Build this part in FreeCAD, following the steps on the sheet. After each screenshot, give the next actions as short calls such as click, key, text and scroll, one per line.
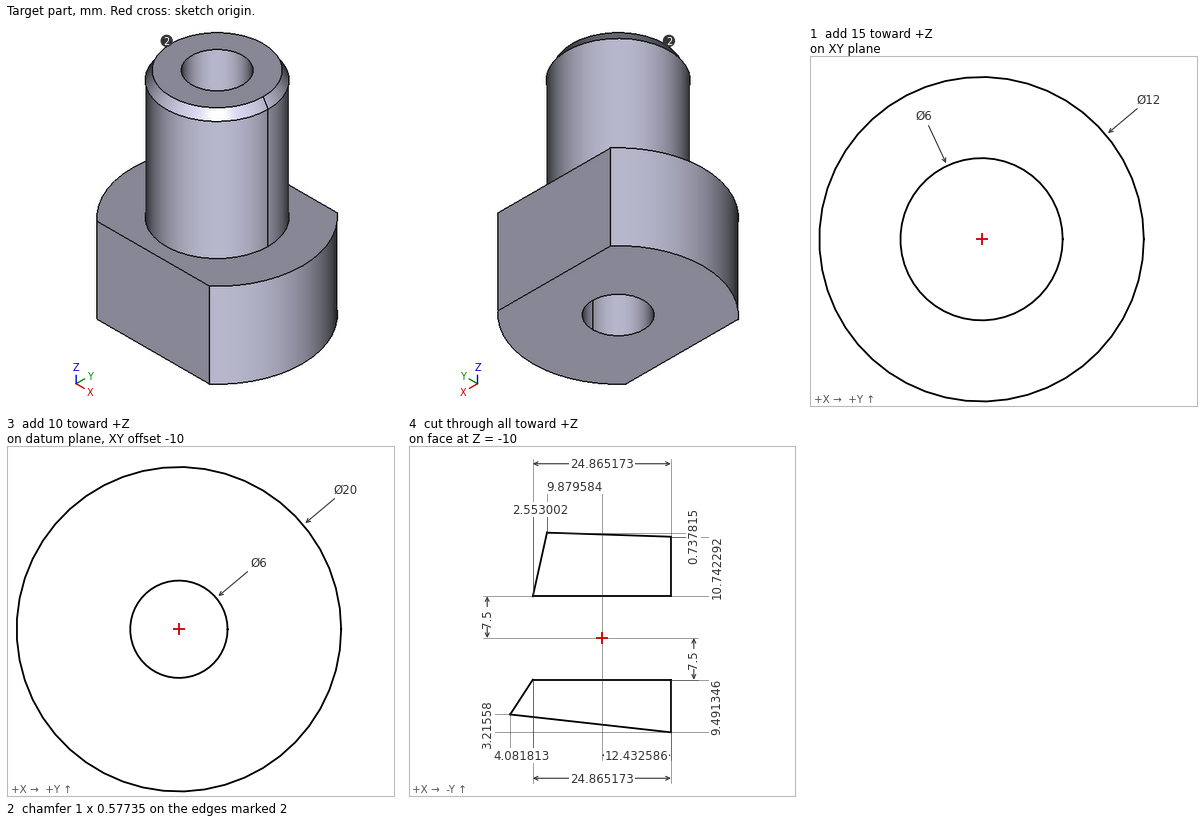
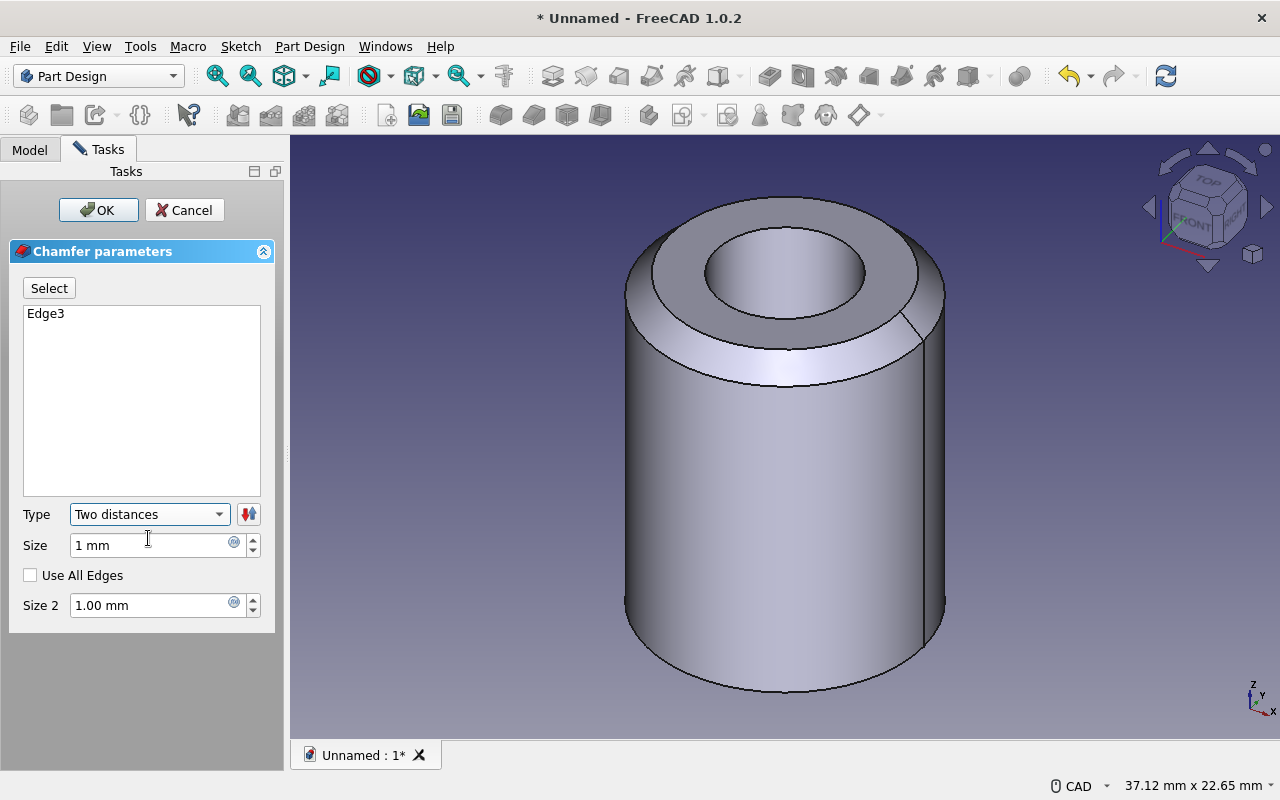
triple_click(158, 606)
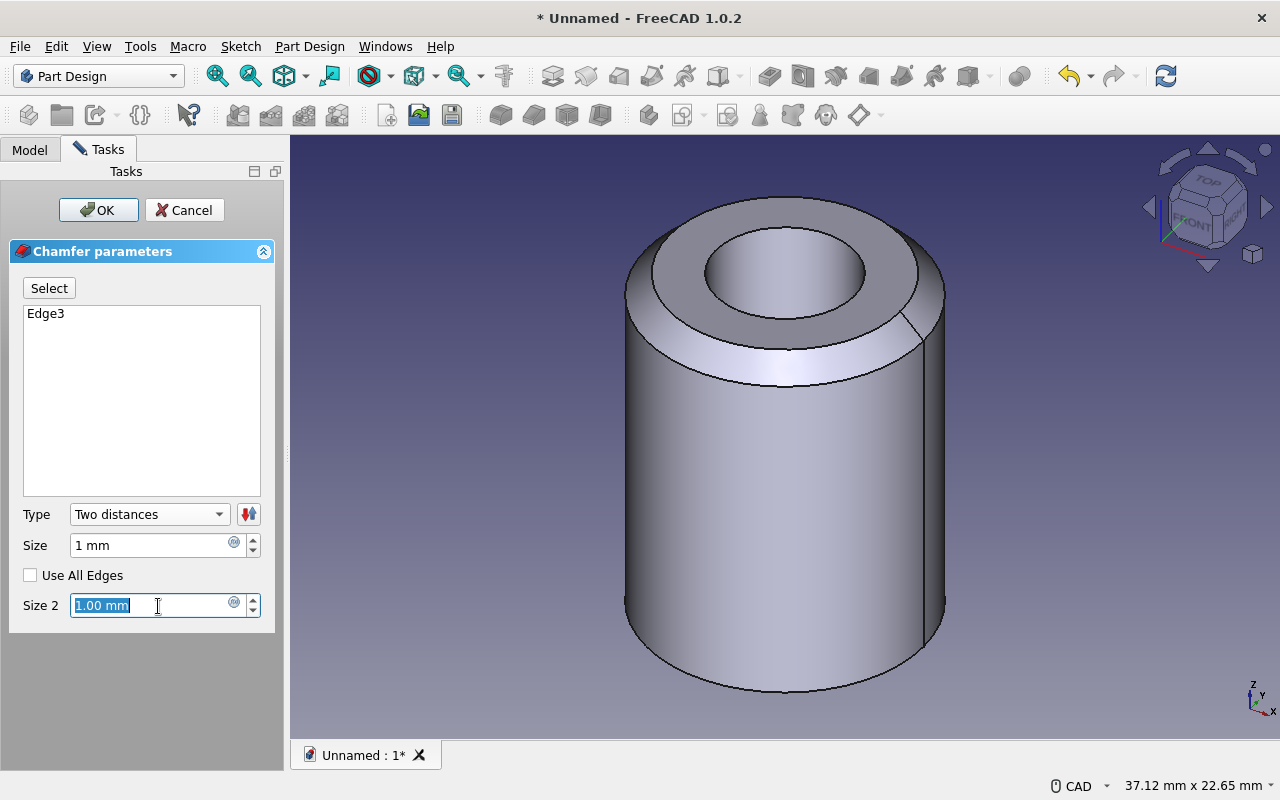
text(0.57735)
key(Tab)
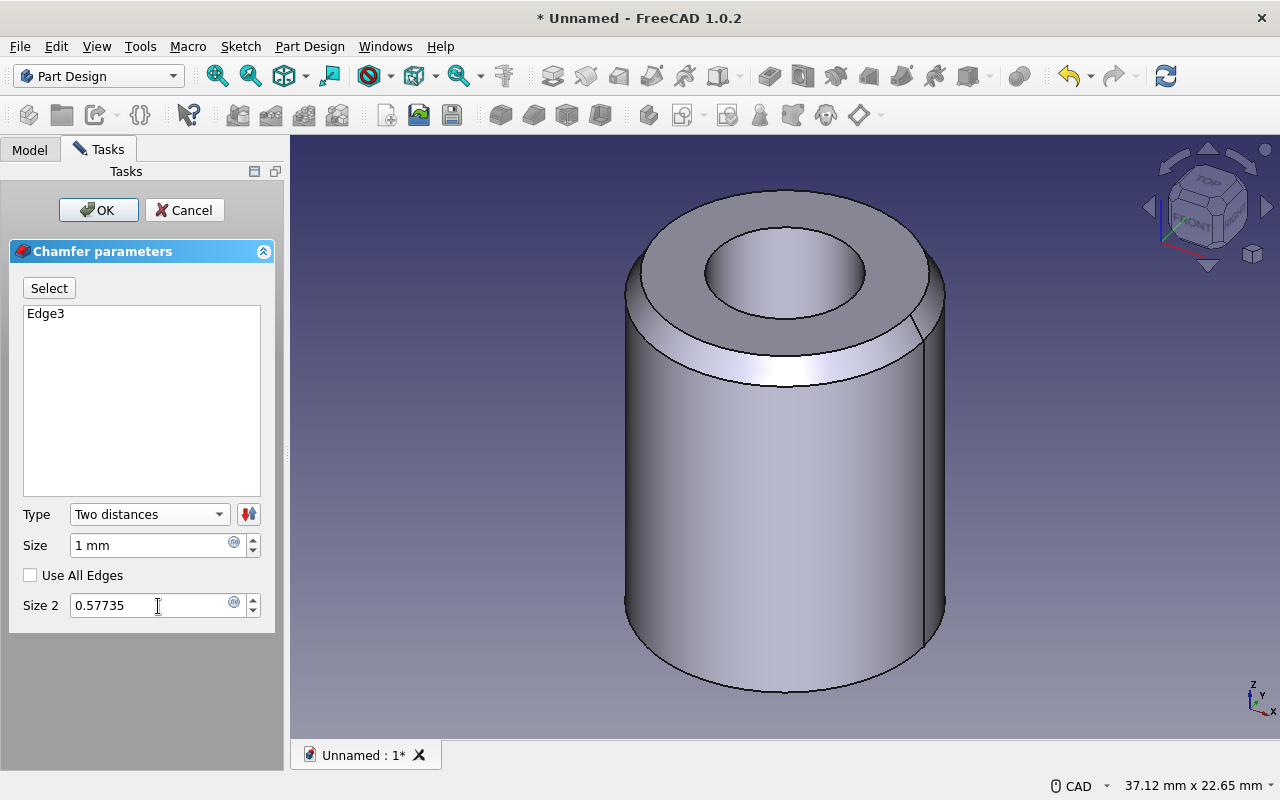
click(99, 210)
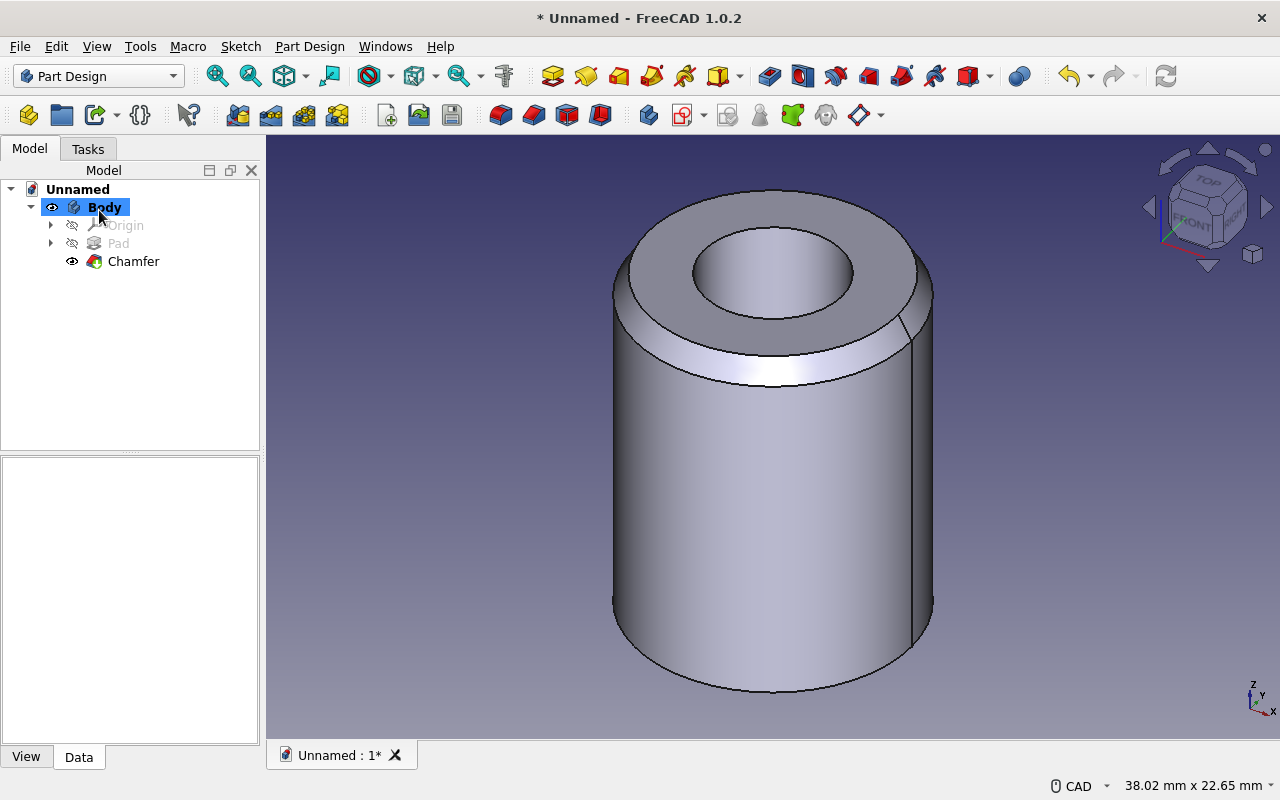
click(51, 225)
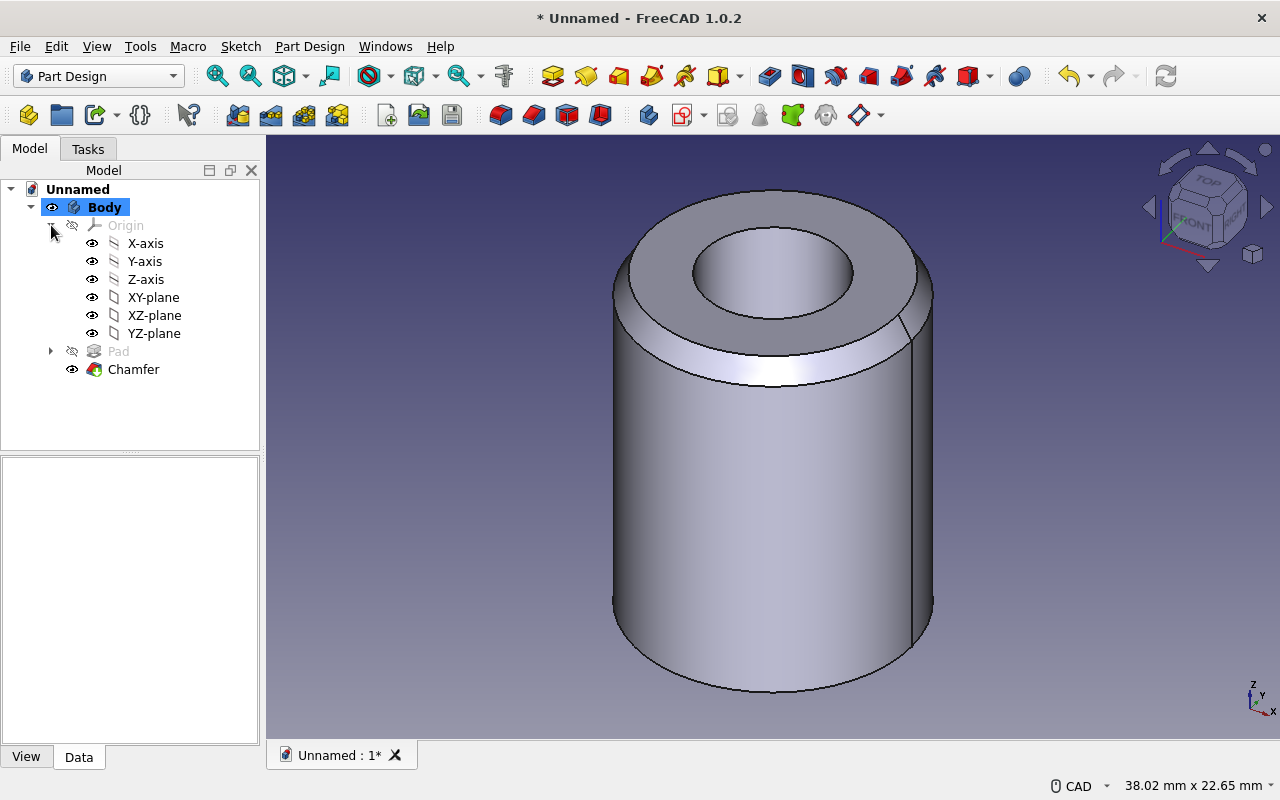
click(137, 297)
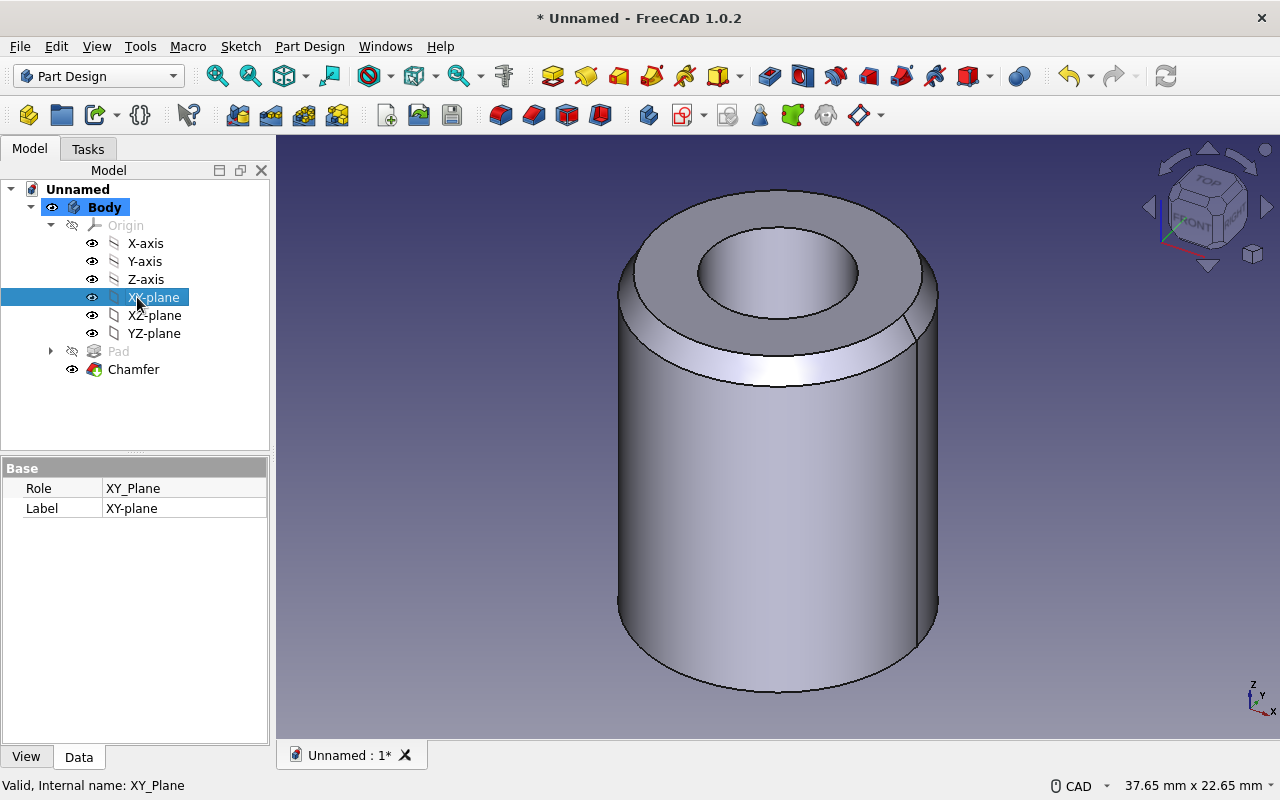
click(858, 116)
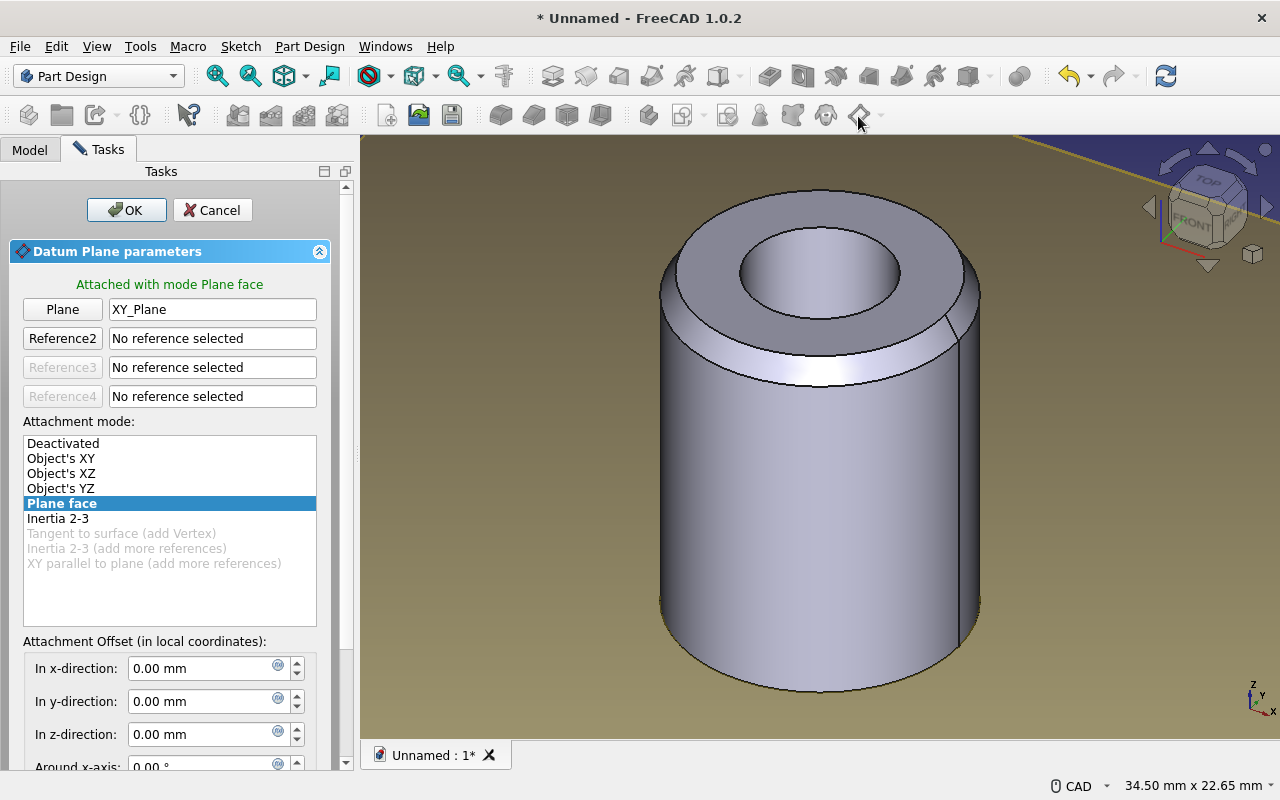
triple_click(210, 734)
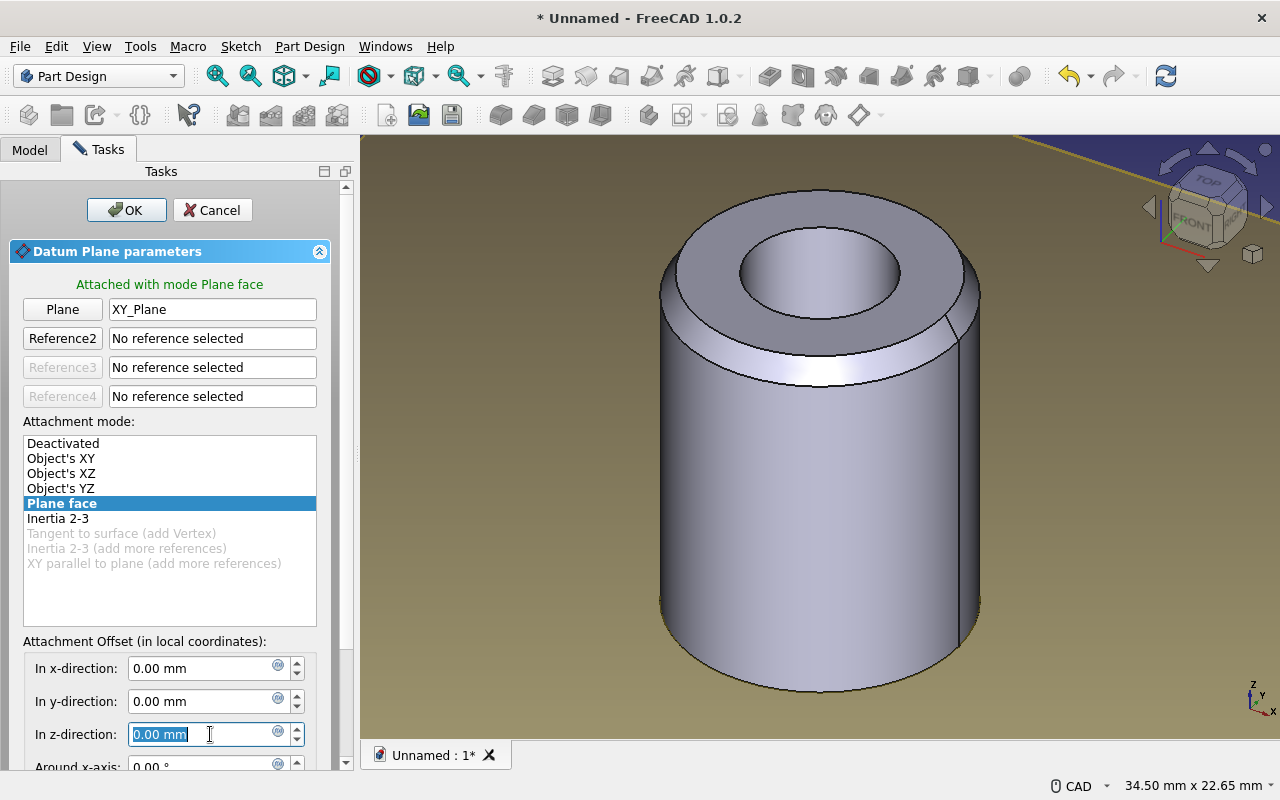
text(-10)
key(Tab)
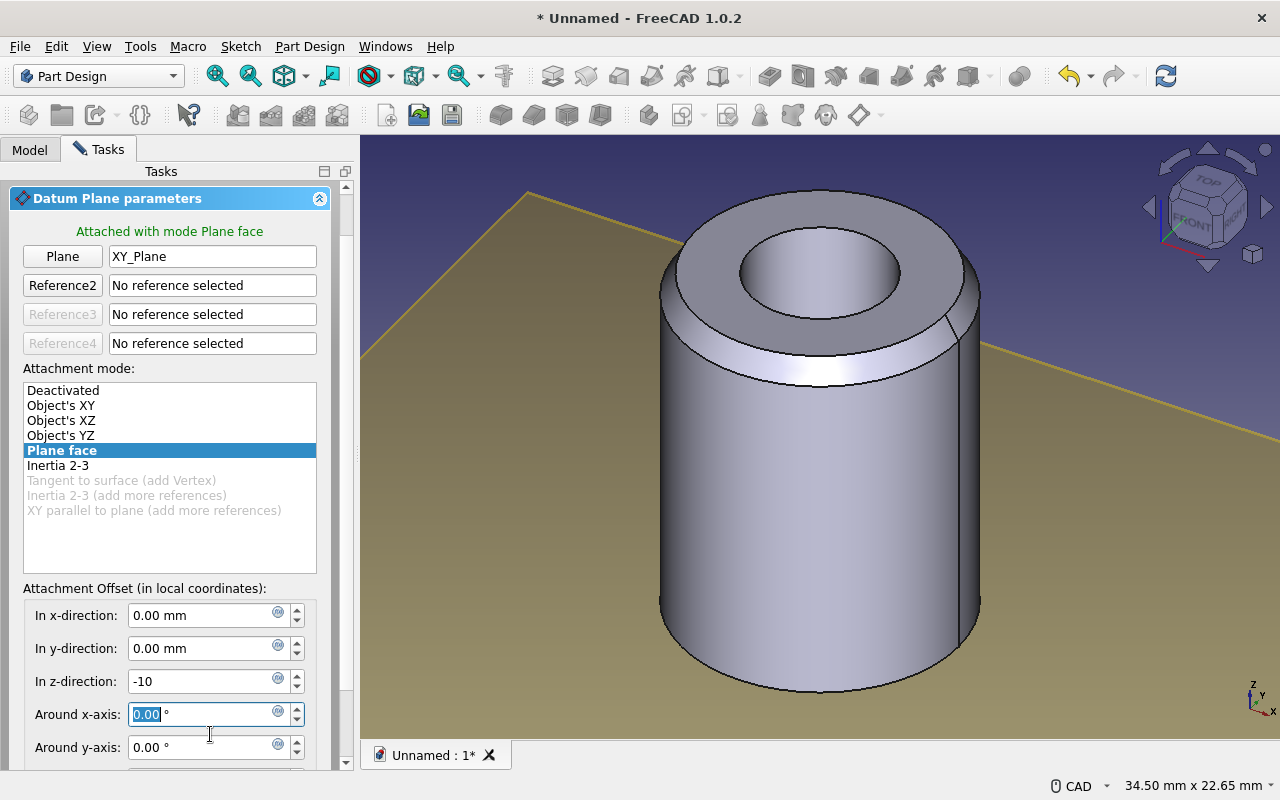
scroll(346, 476, up, 2)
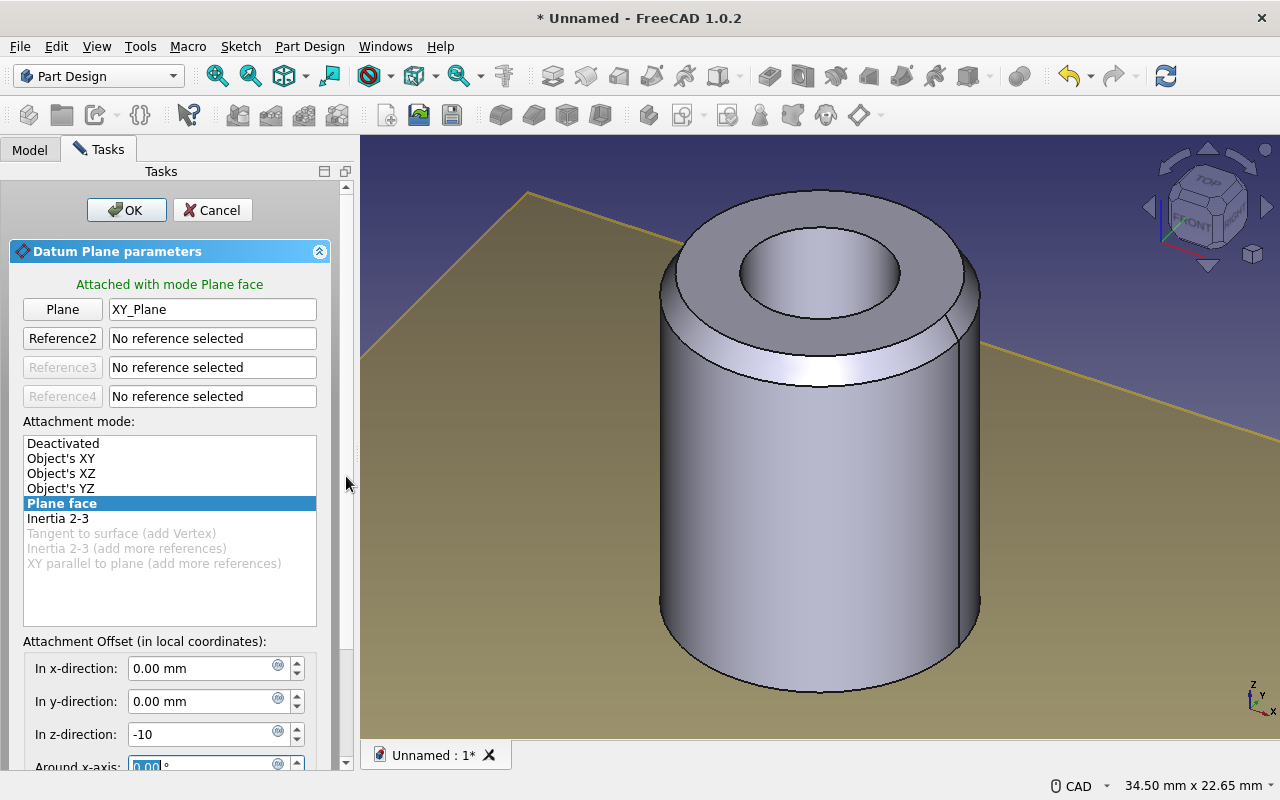
click(127, 210)